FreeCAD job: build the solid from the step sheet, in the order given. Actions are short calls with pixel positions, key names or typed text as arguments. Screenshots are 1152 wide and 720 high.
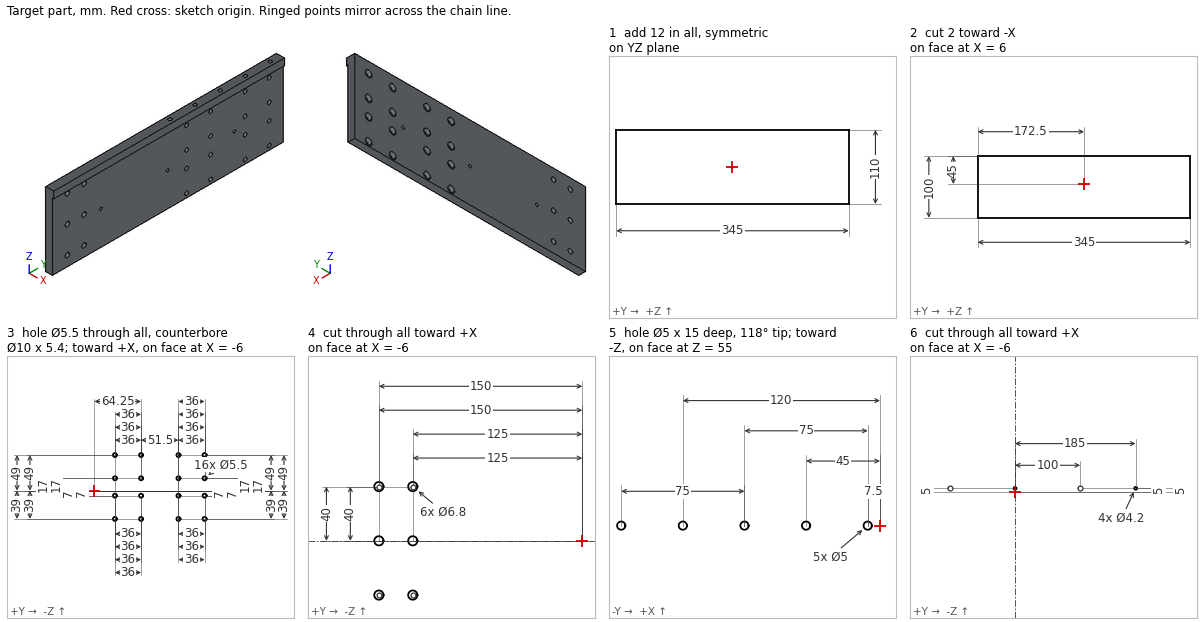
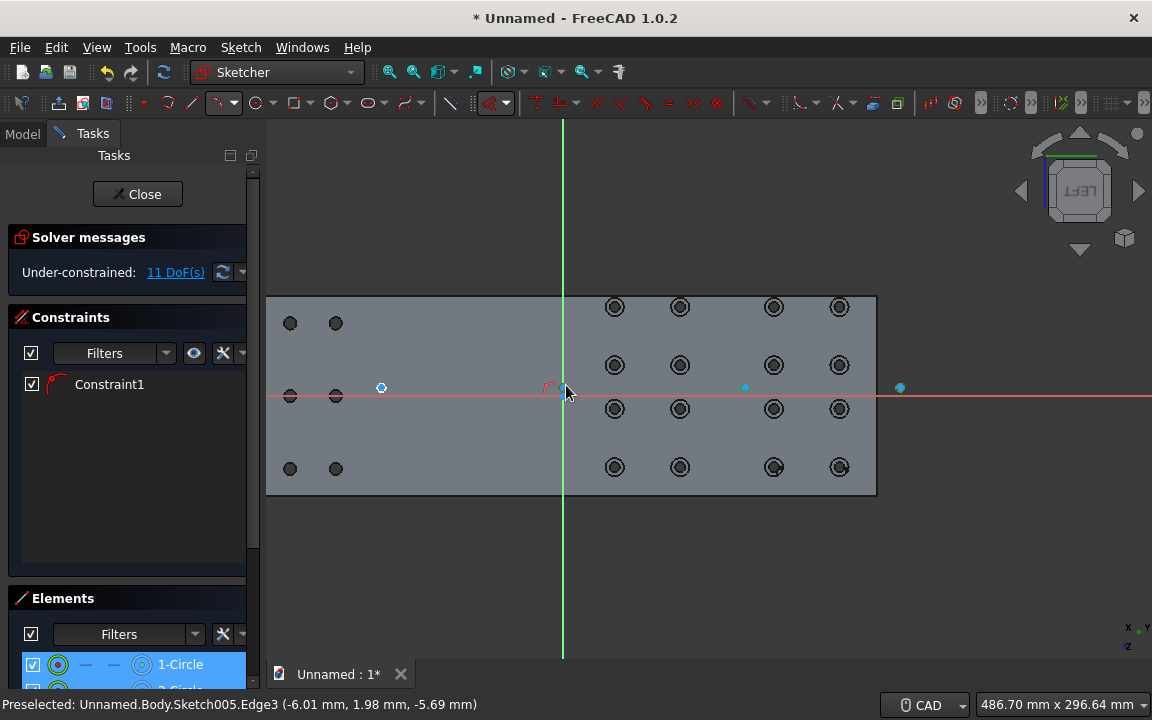
scroll(384, 385, up, 7)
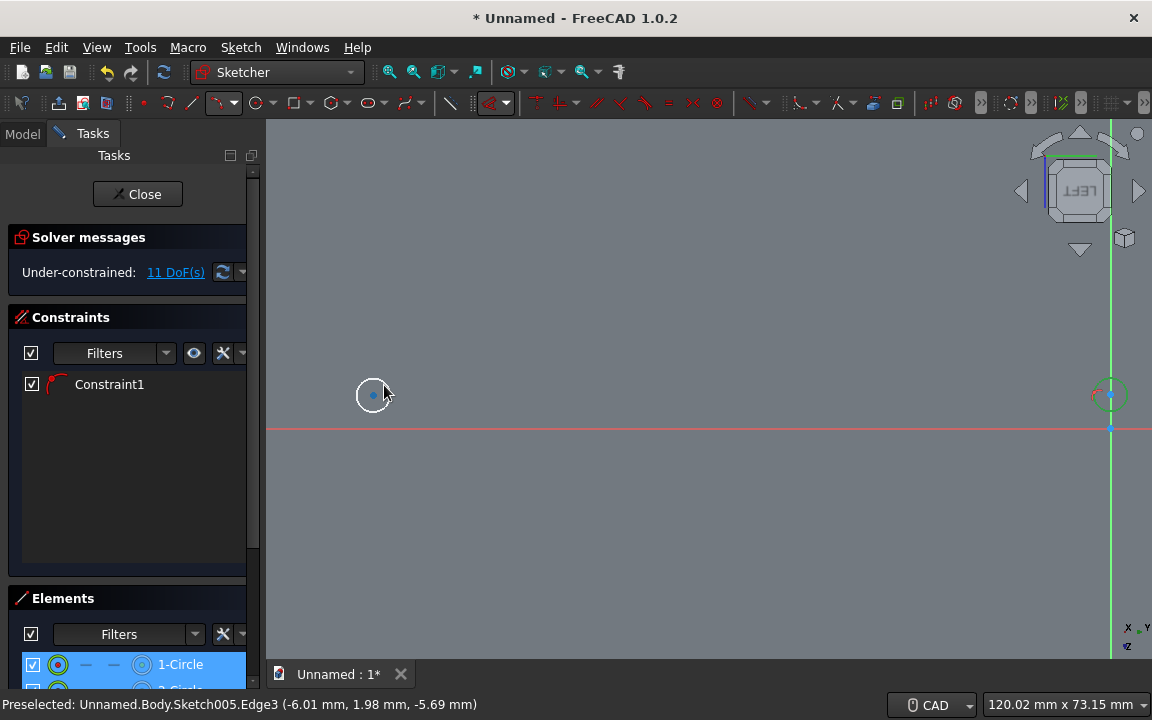
click(385, 383)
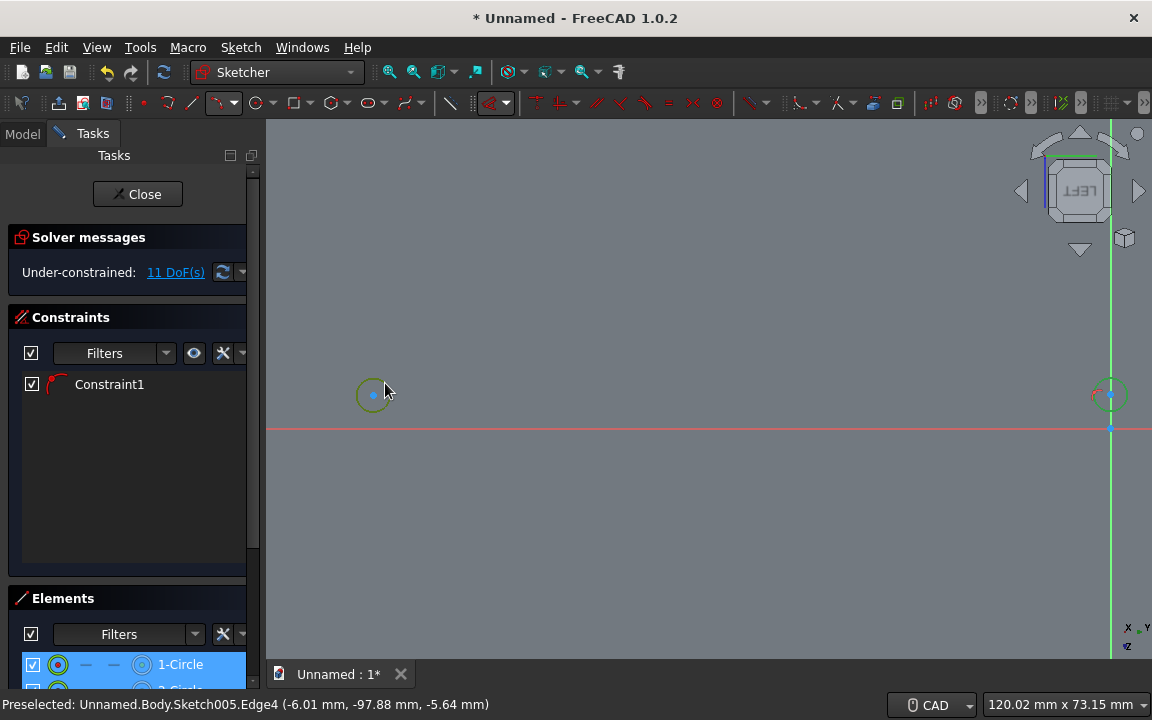
click(670, 104)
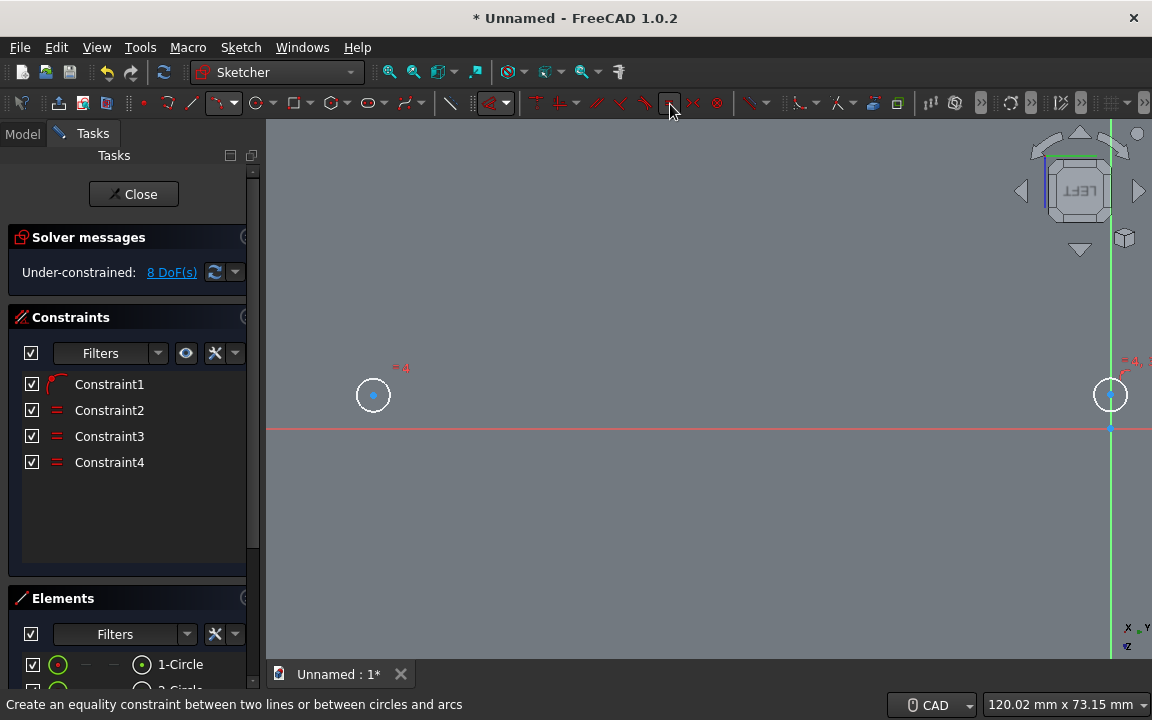
scroll(384, 385, down, 7)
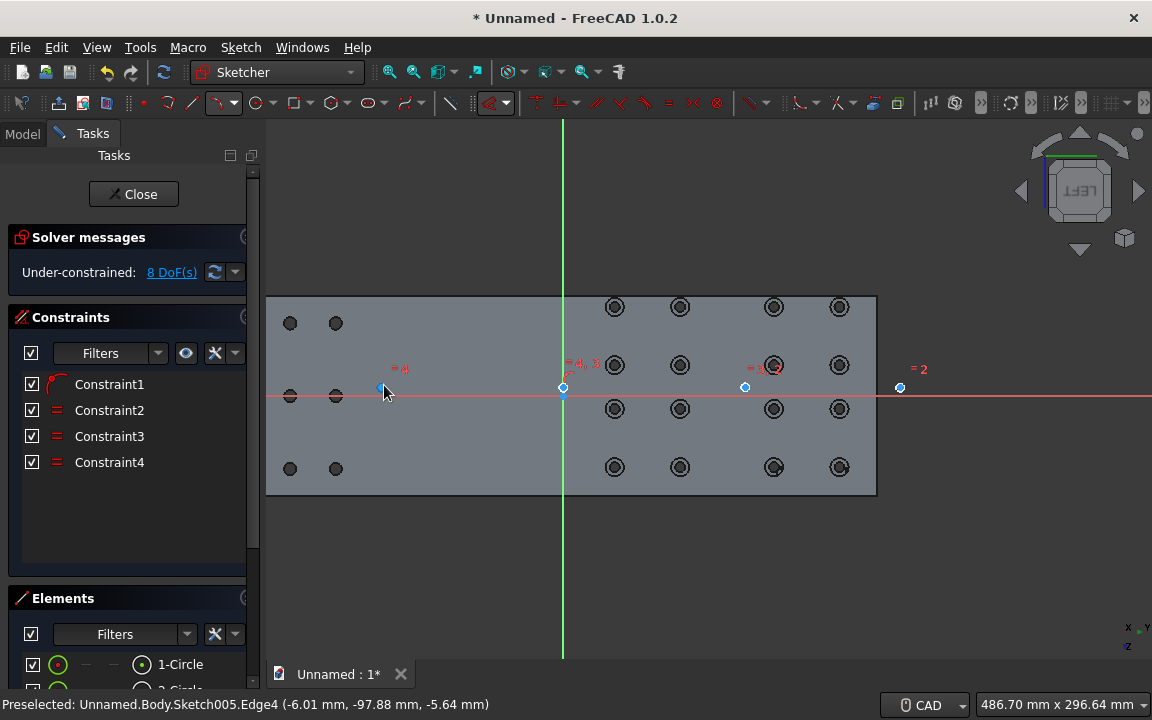
click(745, 387)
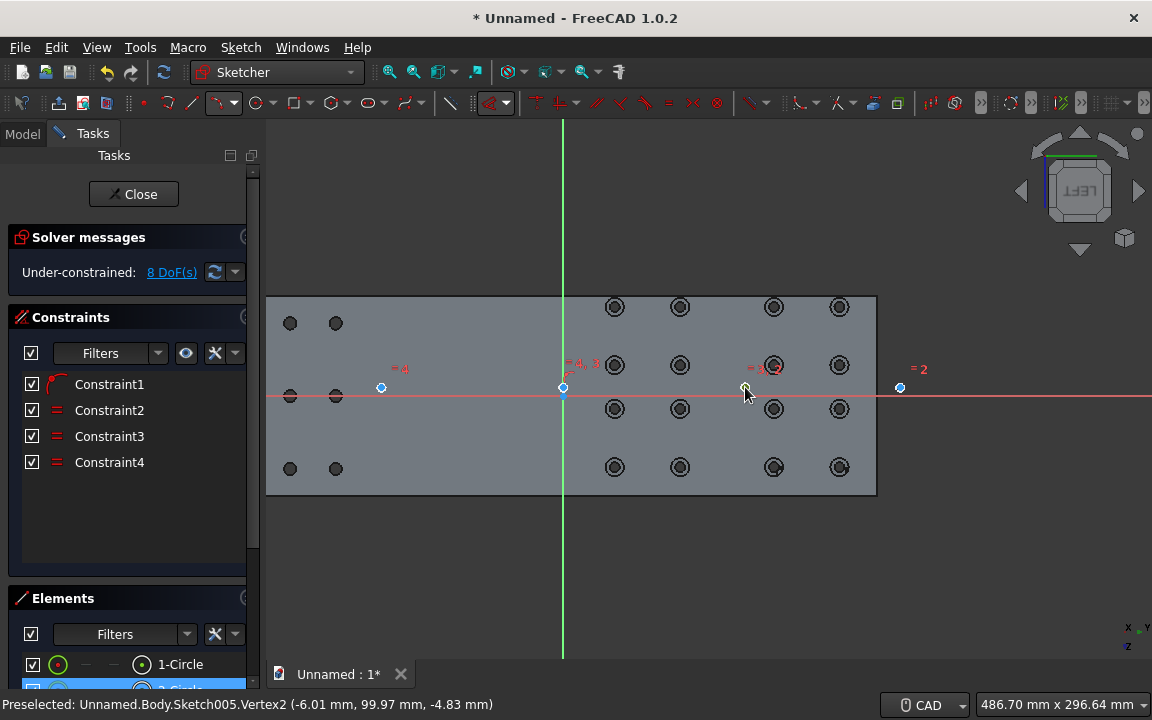
click(381, 388)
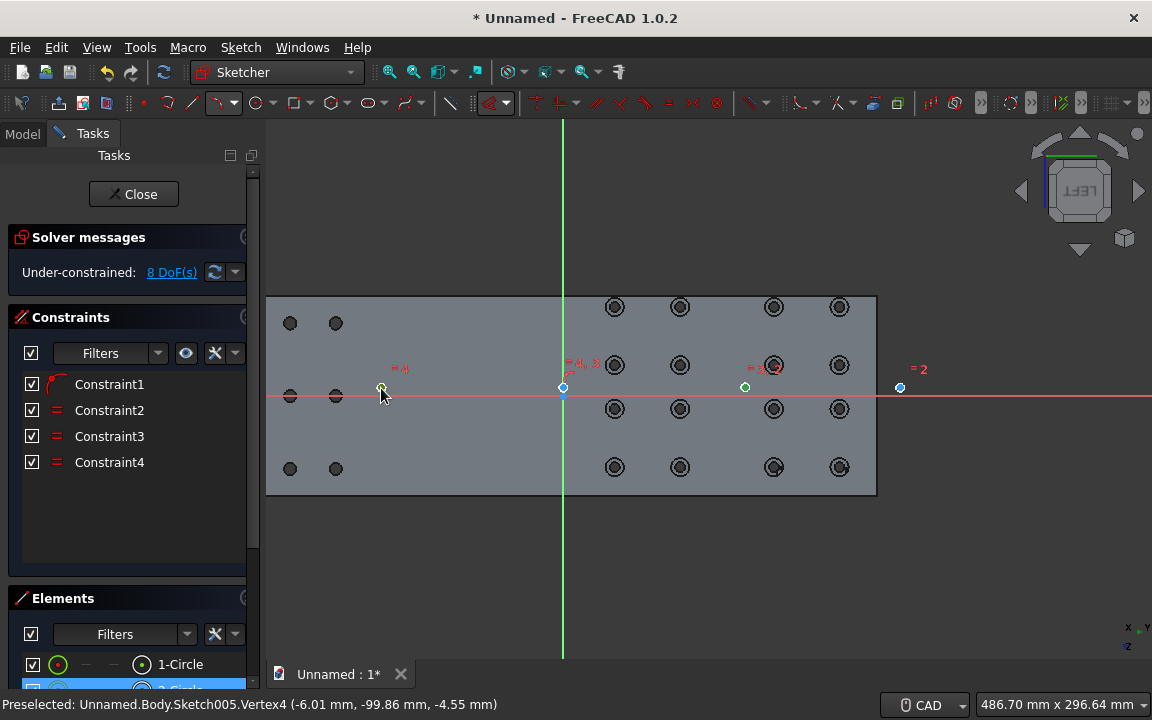
click(563, 596)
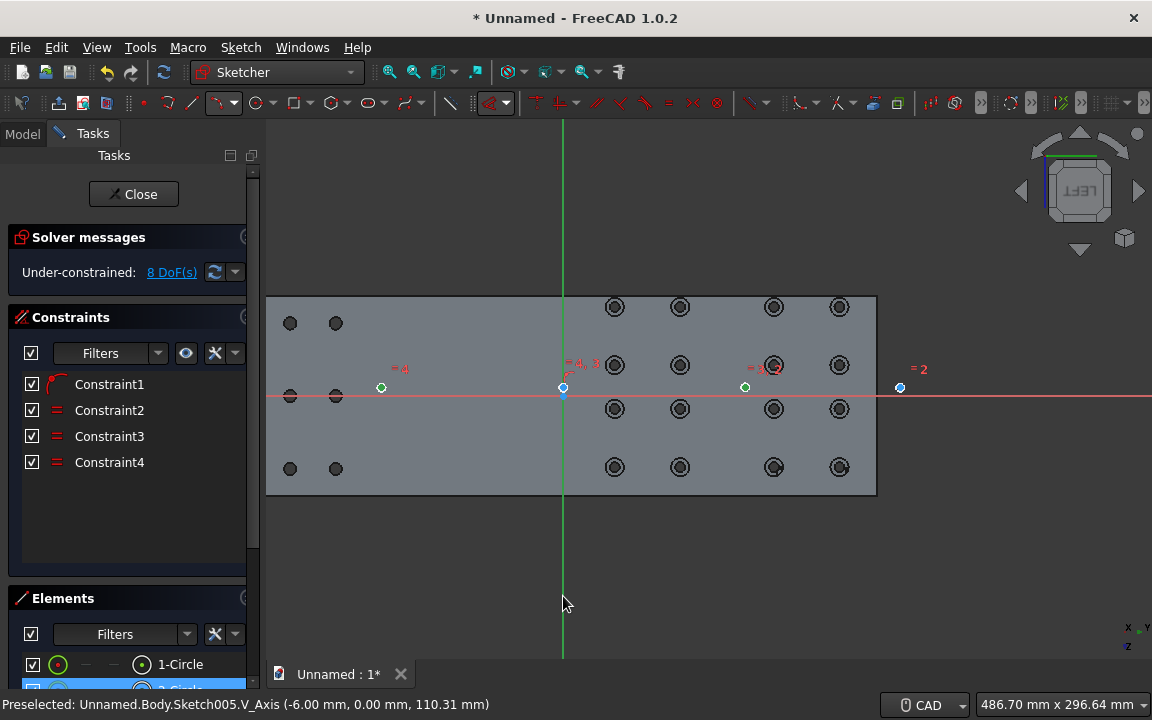
click(694, 104)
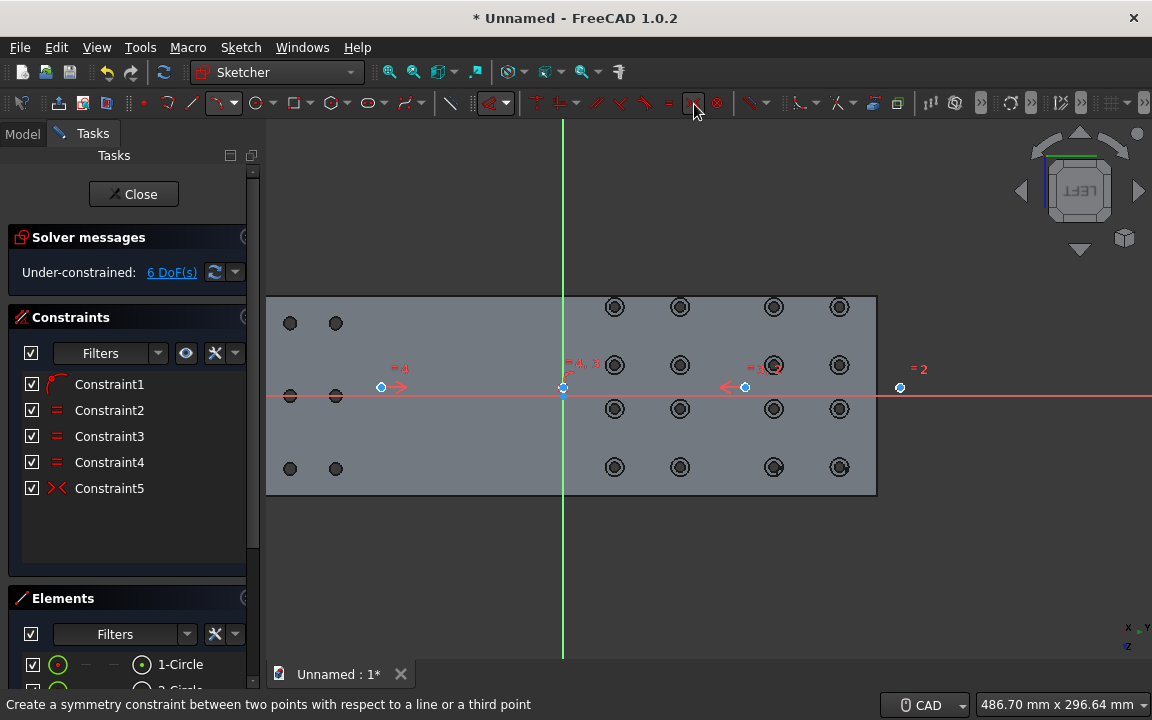
scroll(904, 388, up, 9)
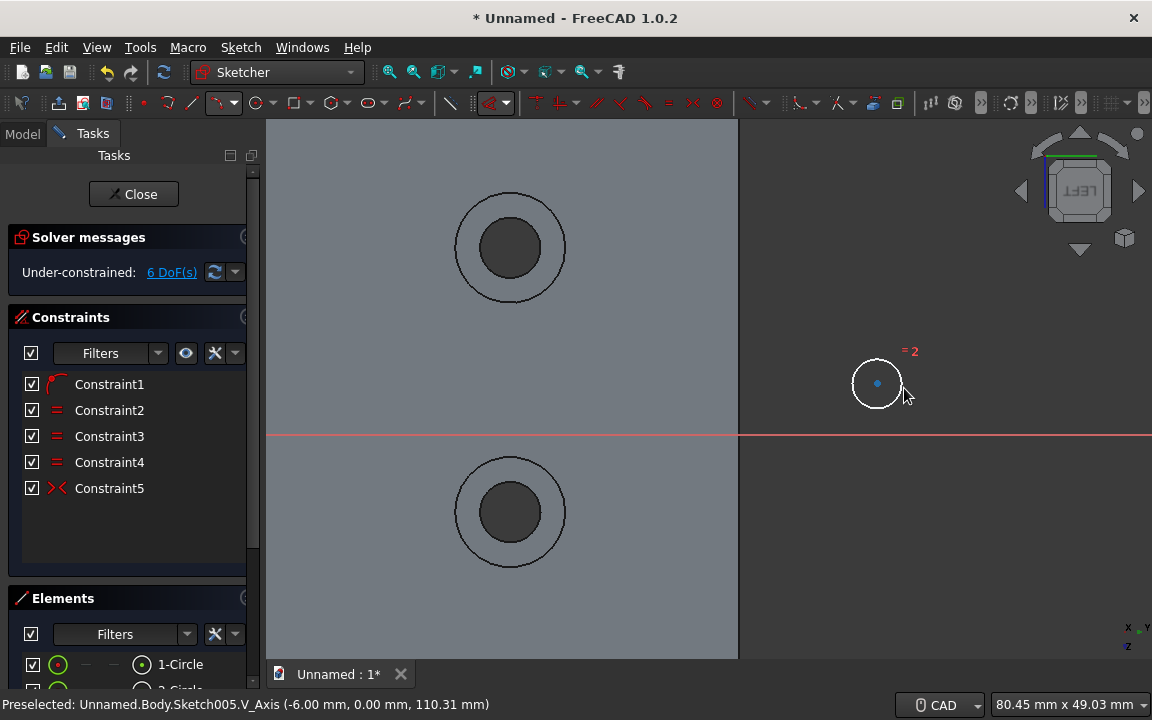
click(902, 385)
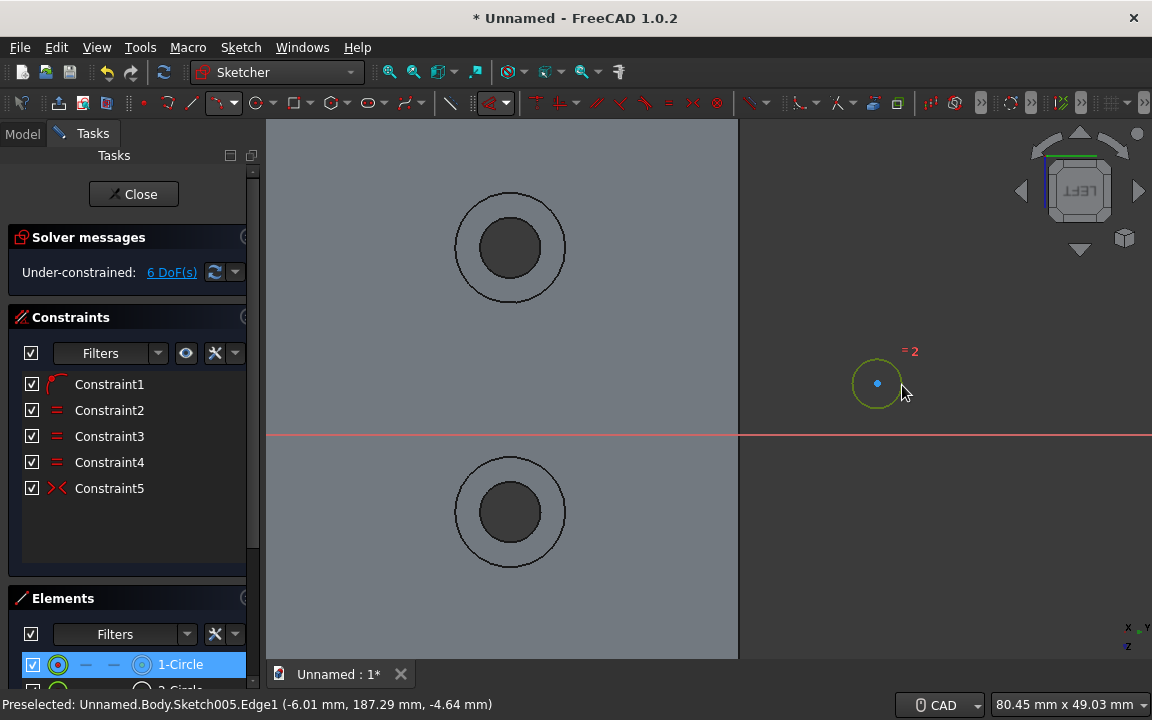
key(k)
key(o)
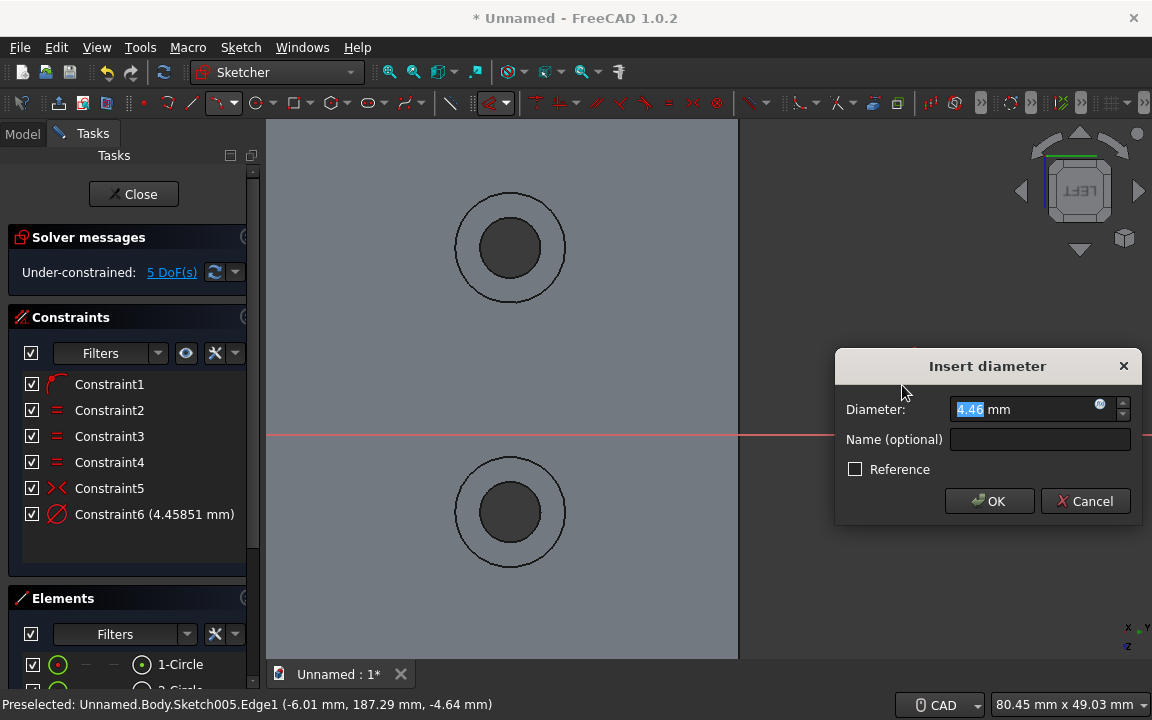
text(4.2)
key(Return)